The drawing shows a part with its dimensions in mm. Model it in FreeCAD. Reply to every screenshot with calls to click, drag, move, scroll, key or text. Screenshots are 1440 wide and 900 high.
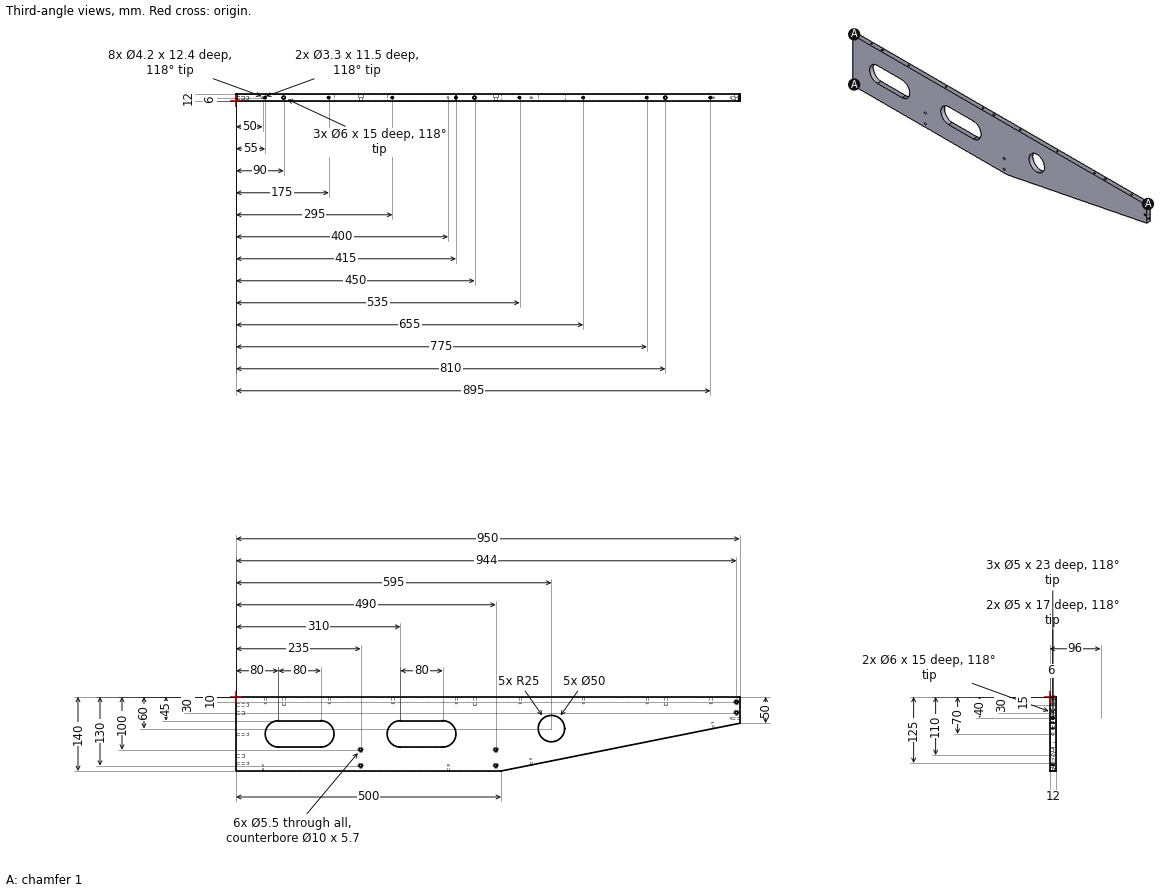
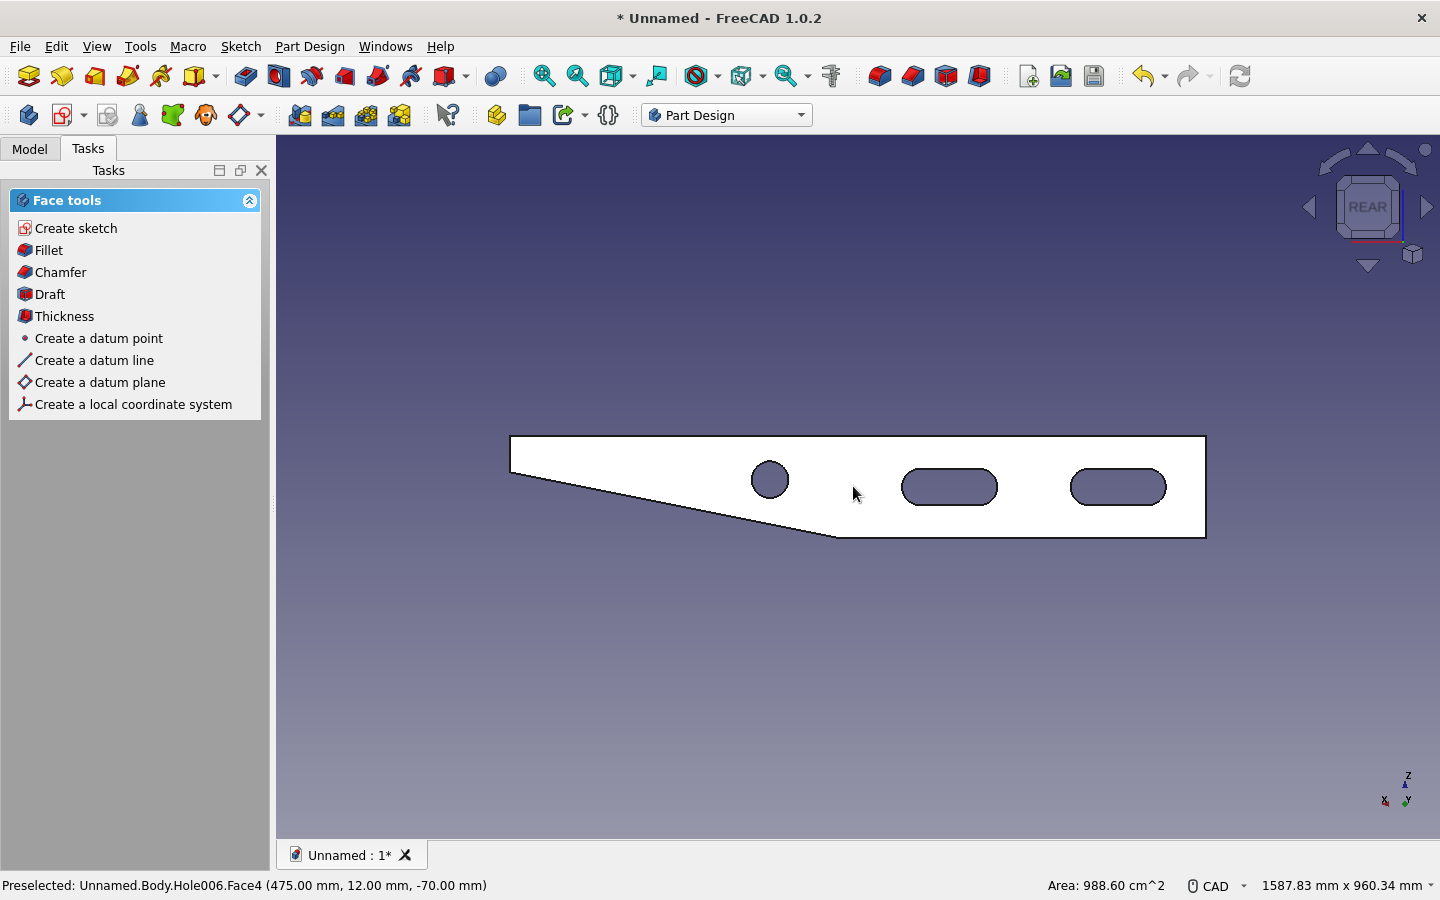
click(62, 116)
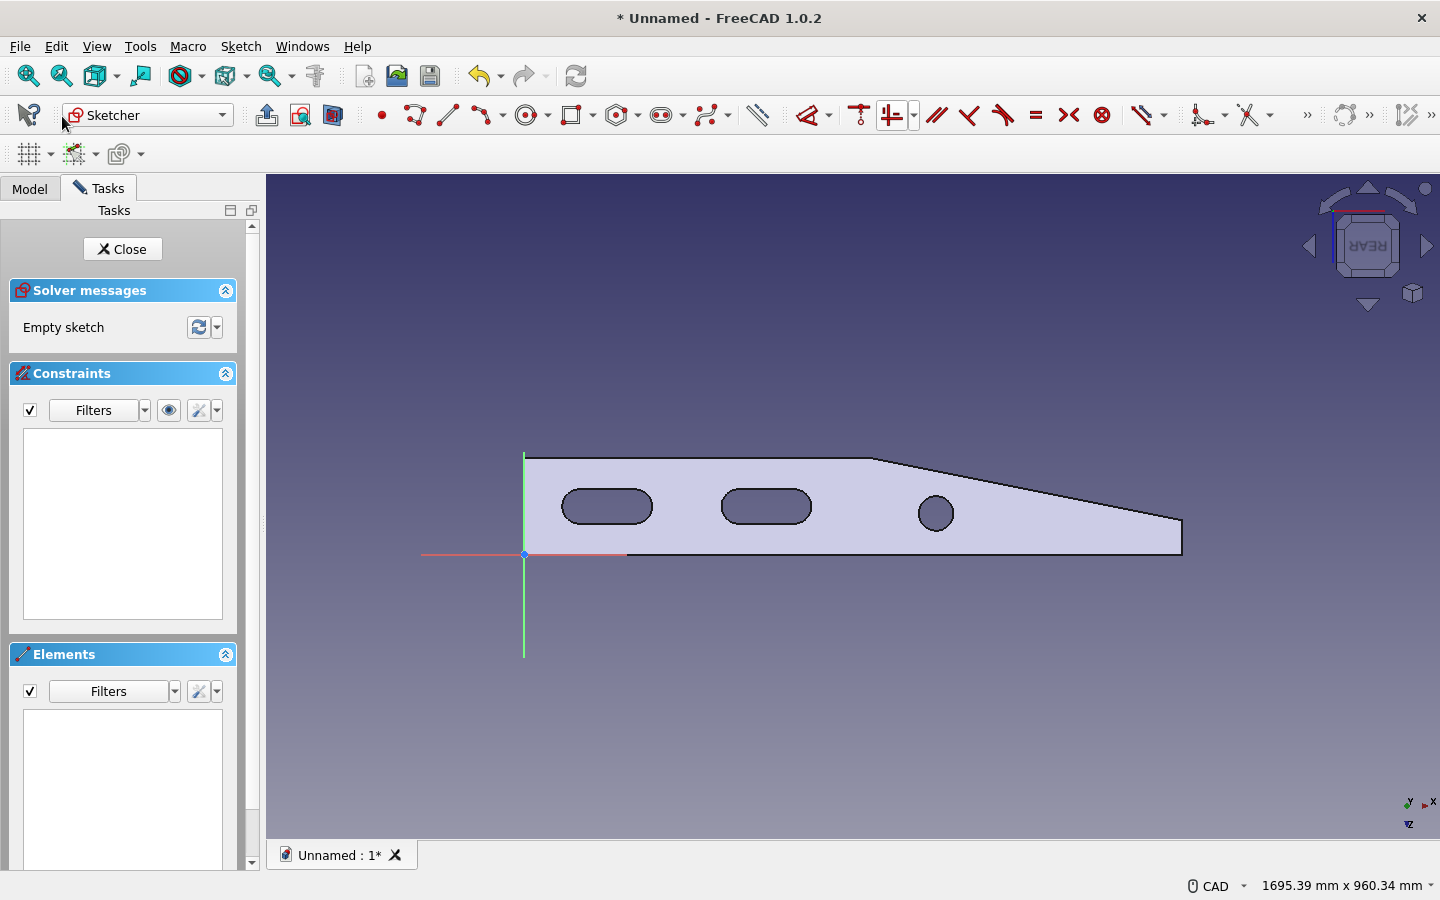
click(526, 116)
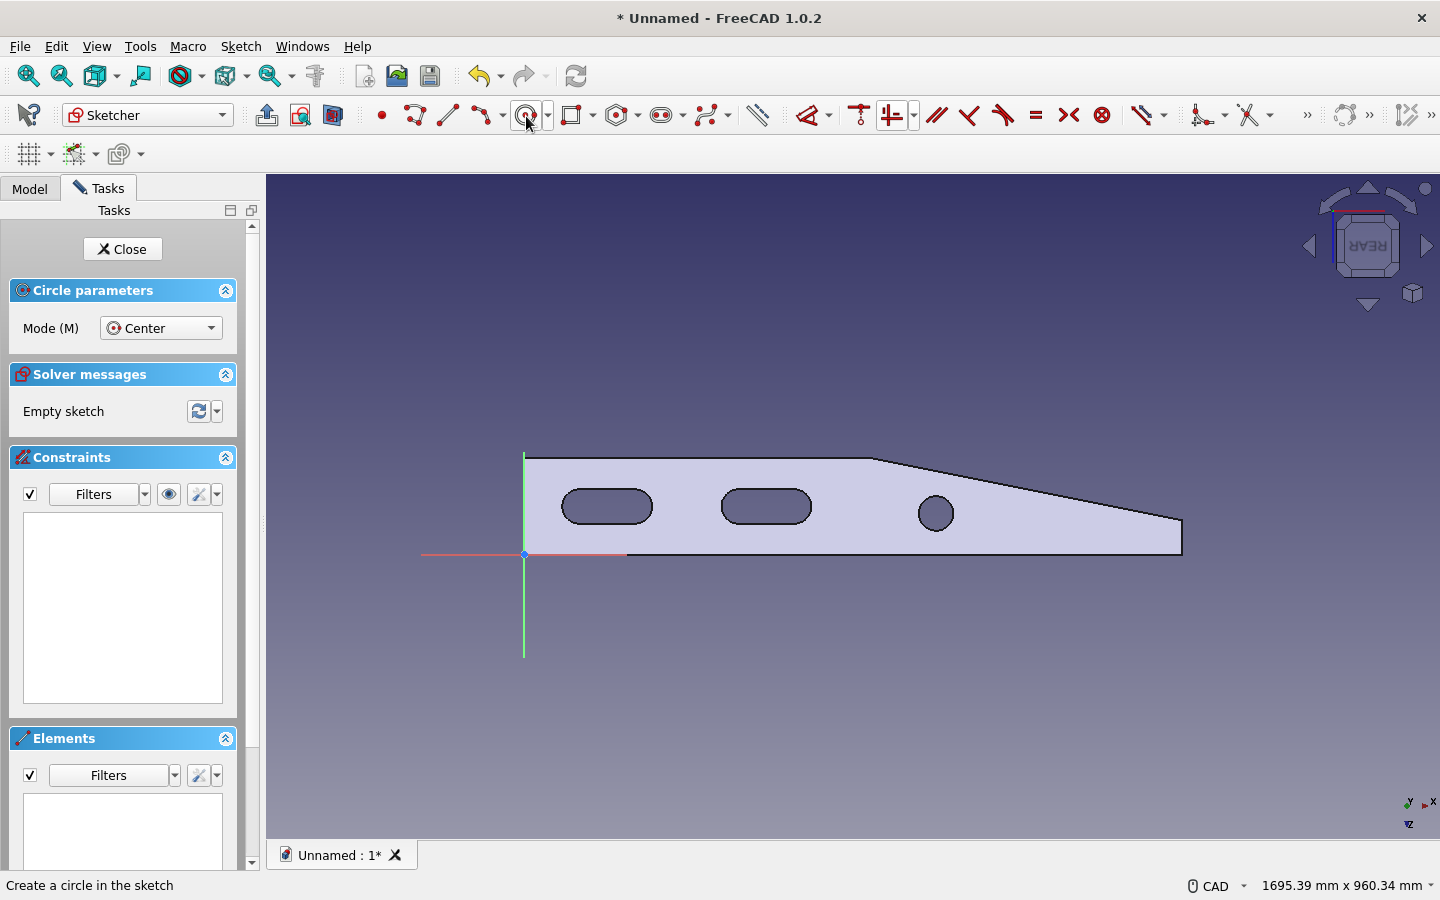
scroll(687, 486, up, 13)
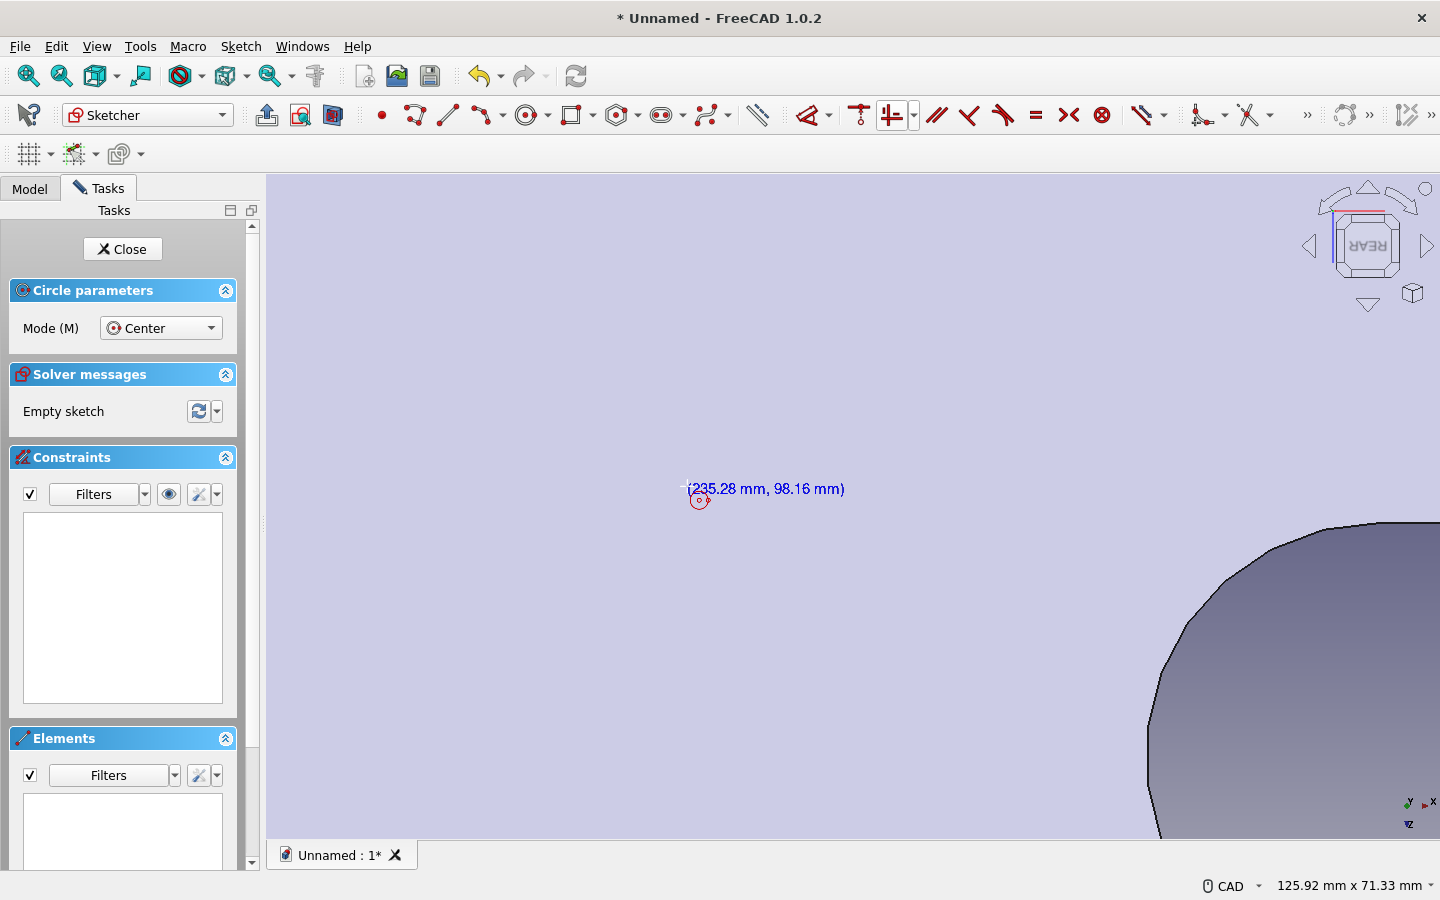
scroll(615, 484, down, 13)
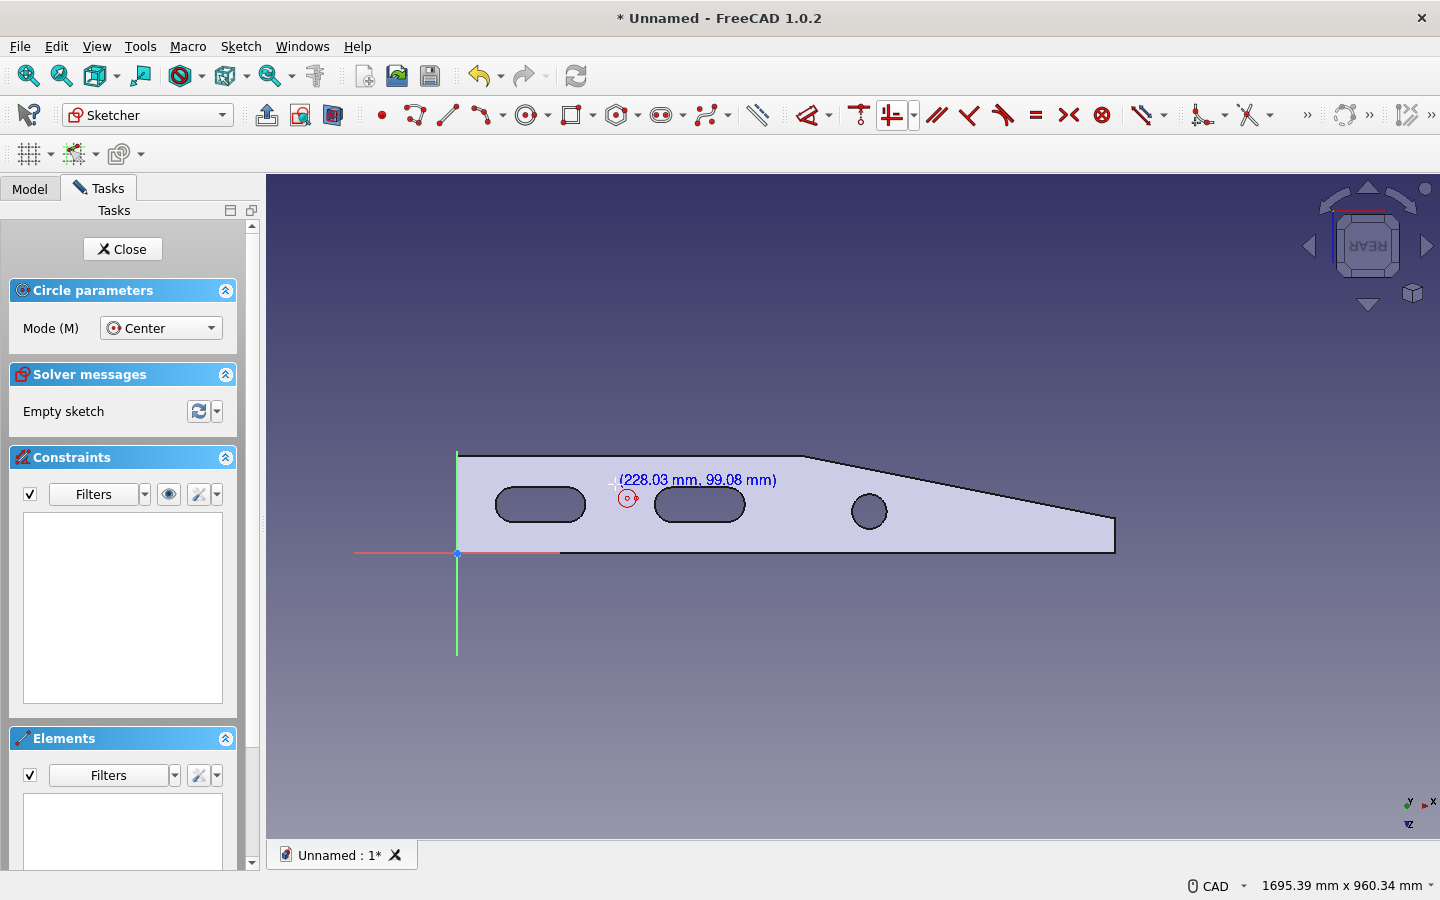
click(620, 484)
move(621, 483)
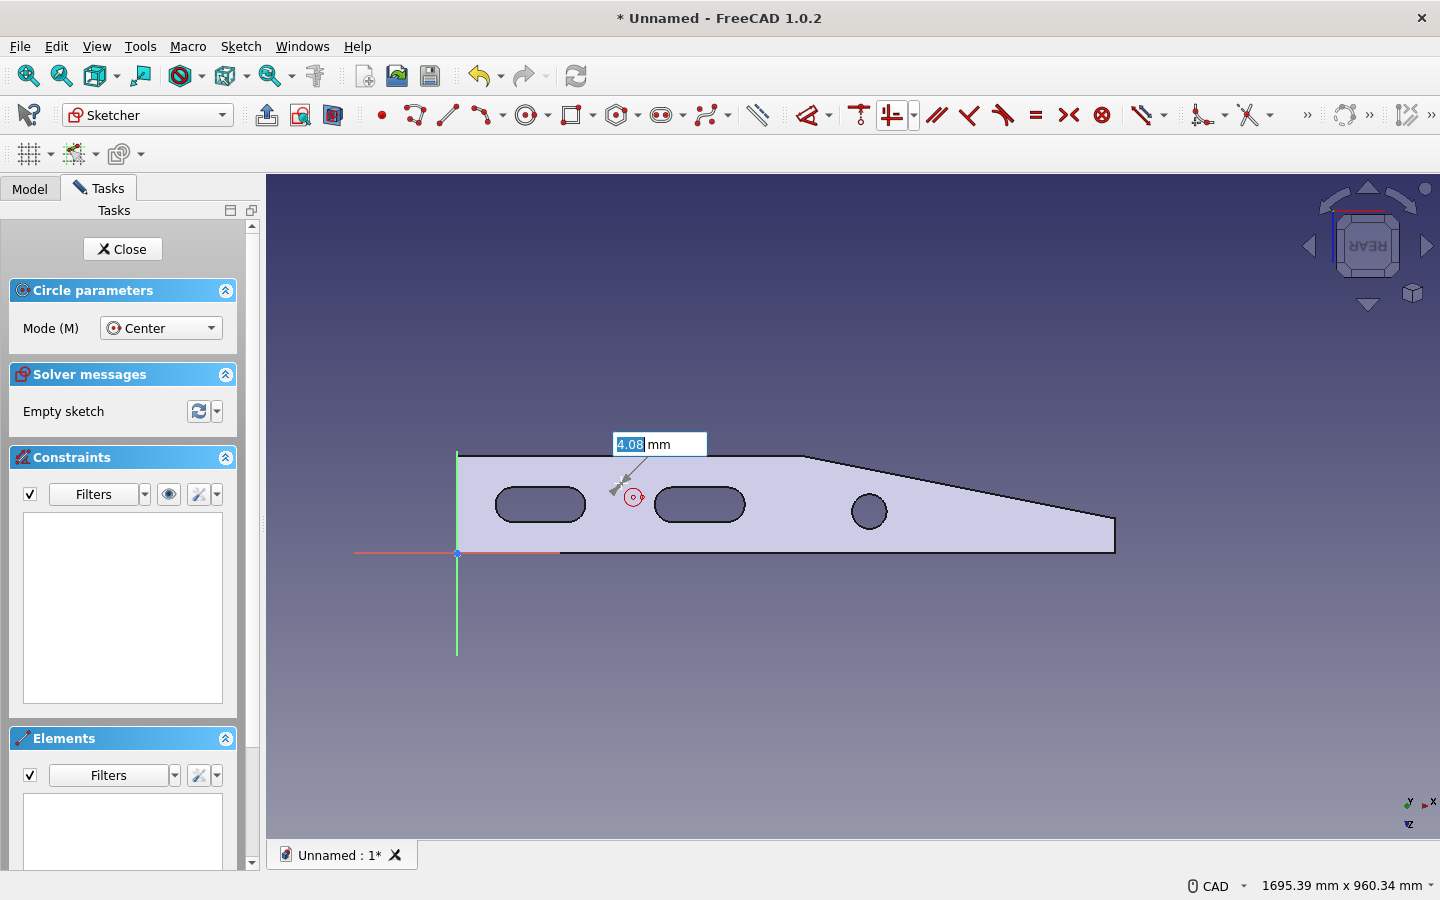
text(5.5)
key(Return)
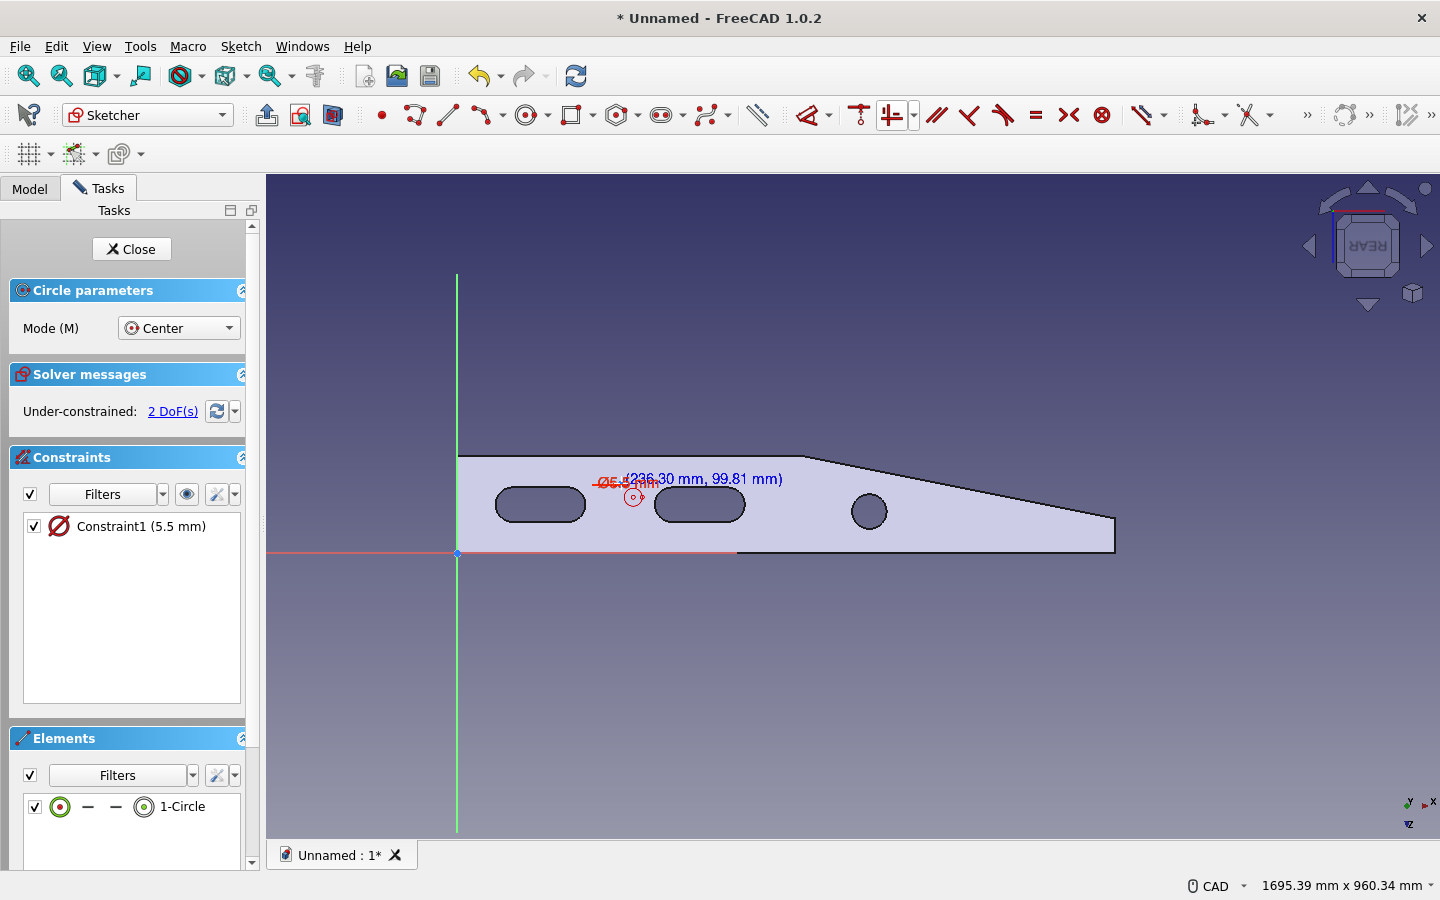
scroll(620, 463, up, 13)